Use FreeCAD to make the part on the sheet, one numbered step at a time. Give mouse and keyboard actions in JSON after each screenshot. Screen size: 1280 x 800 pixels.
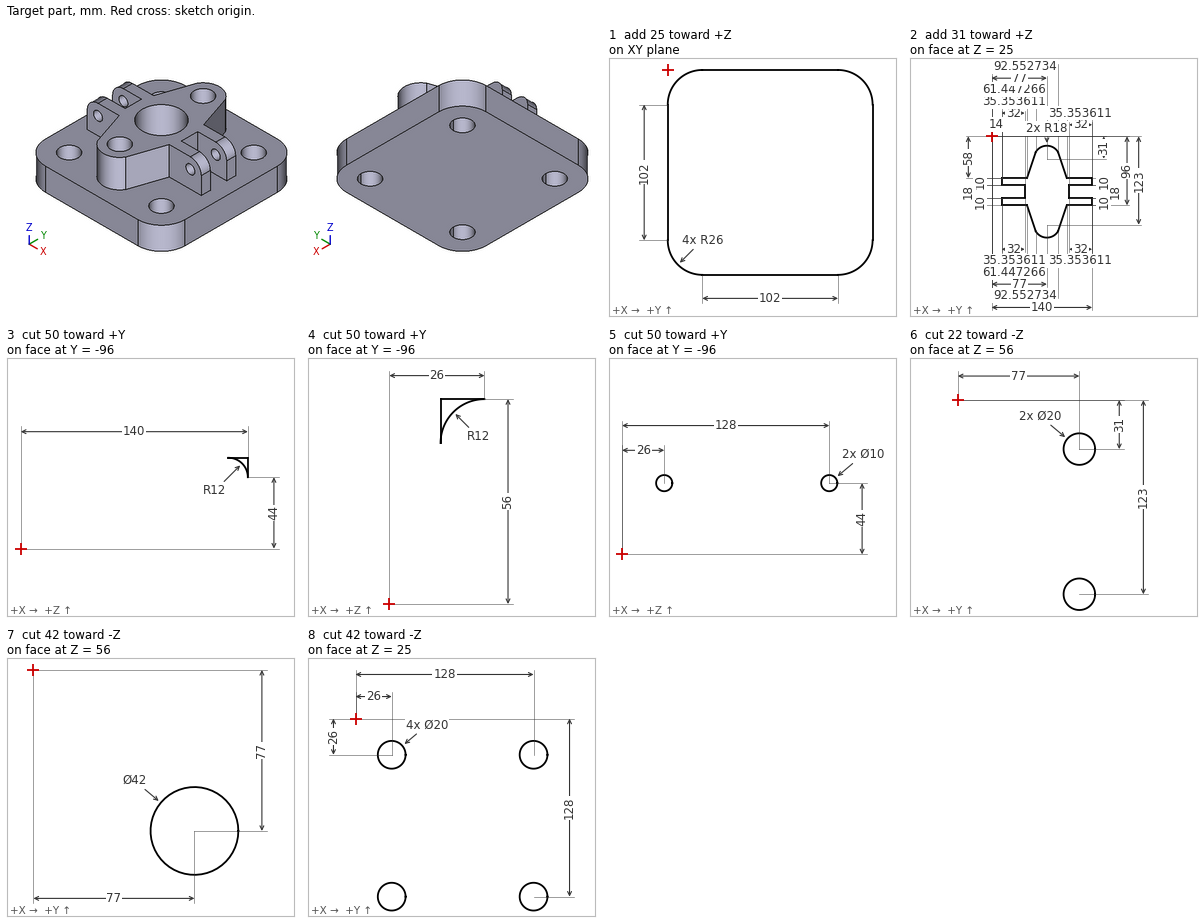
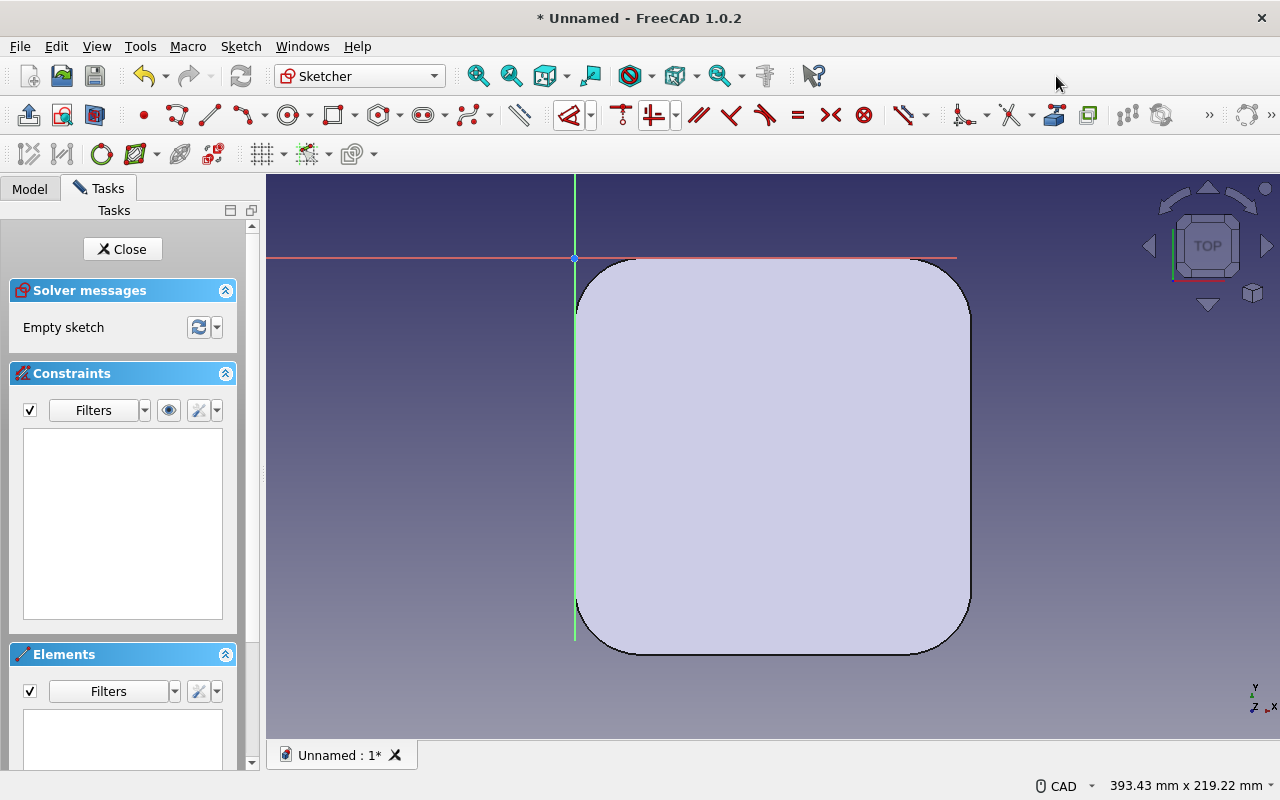
{"action": "left_click", "coordinate": [177, 116]}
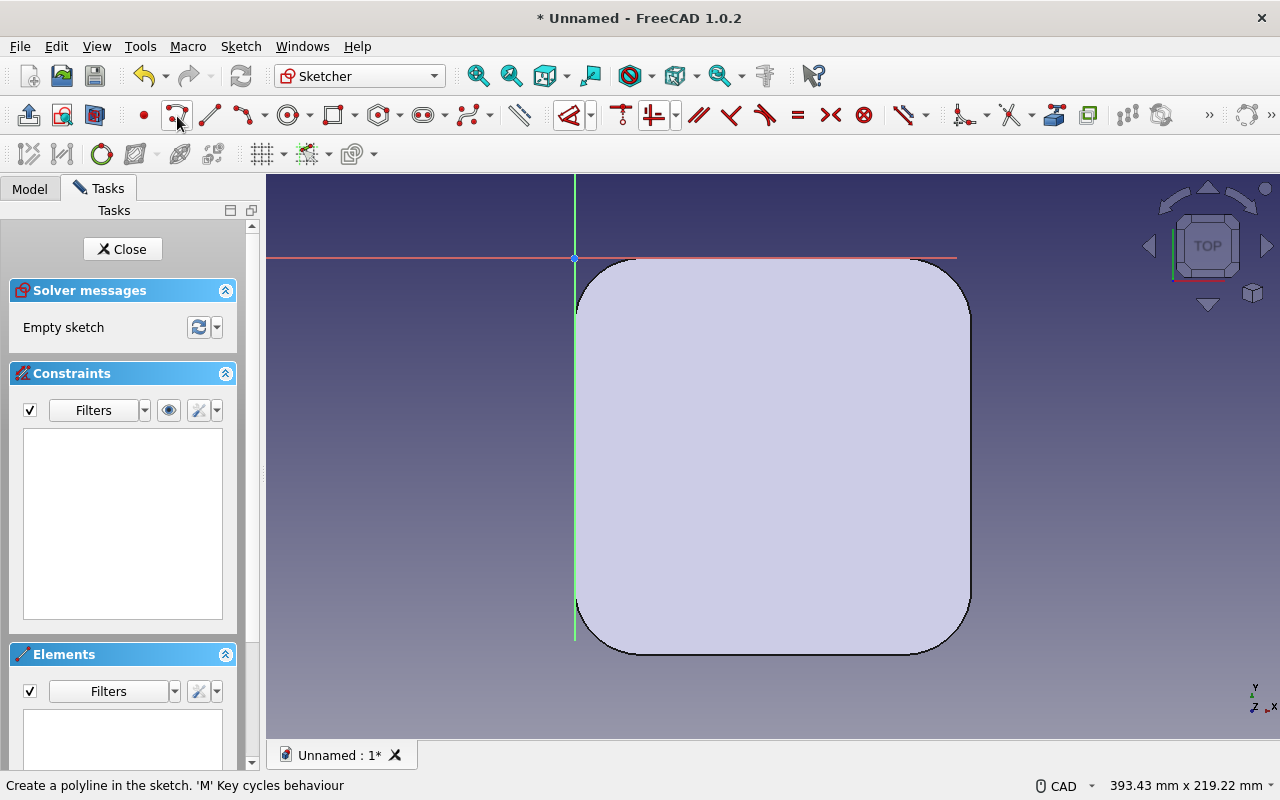
{"action": "left_click", "coordinate": [813, 598]}
{"action": "left_click", "coordinate": [844, 505]}
{"action": "left_click", "coordinate": [935, 505]}
{"action": "left_click", "coordinate": [935, 480]}
{"action": "left_click", "coordinate": [853, 480]}
{"action": "left_click", "coordinate": [853, 433]}
{"action": "left_click", "coordinate": [935, 433]}
{"action": "left_click", "coordinate": [935, 408]}
{"action": "left_click", "coordinate": [844, 408]}
{"action": "left_click", "coordinate": [813, 315]}
{"action": "right_click", "coordinate": [813, 315]}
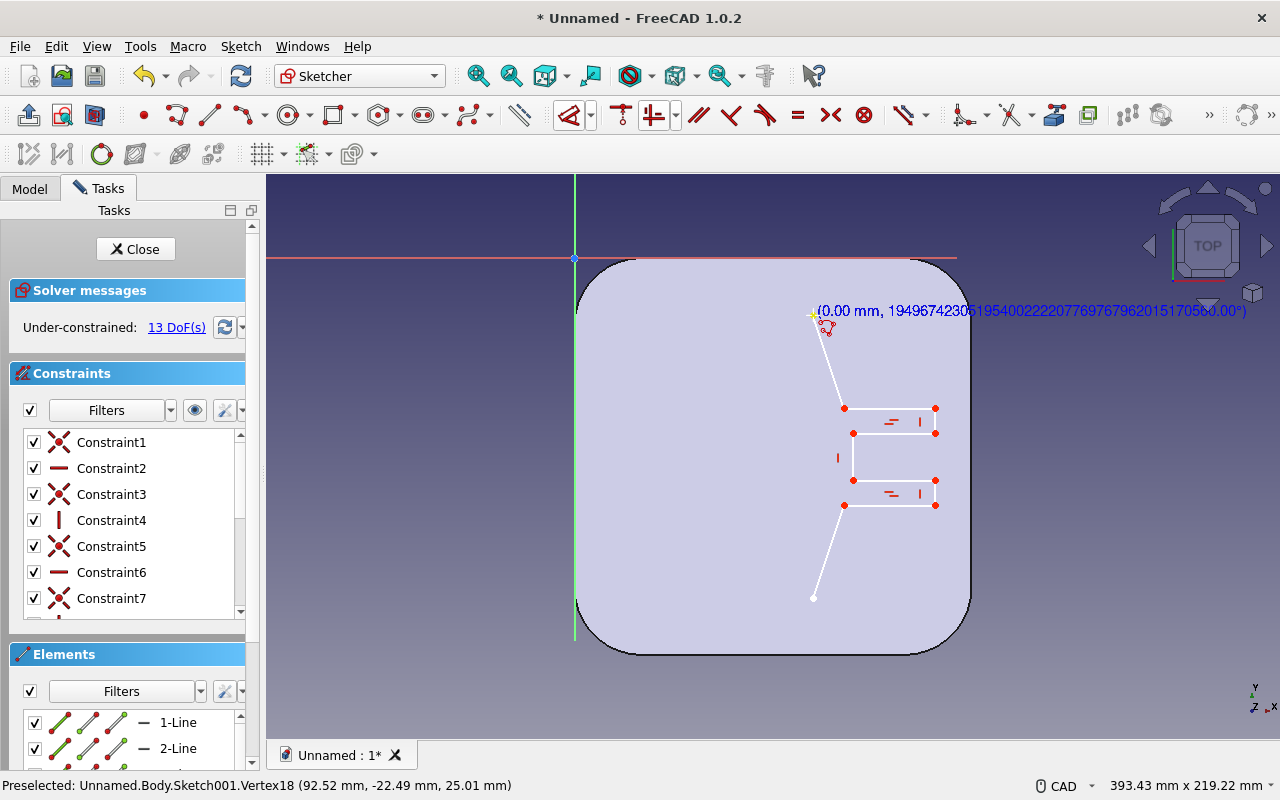
{"action": "left_click", "coordinate": [733, 315]}
{"action": "left_click", "coordinate": [702, 408]}
{"action": "left_click", "coordinate": [611, 408]}
{"action": "left_click", "coordinate": [611, 433]}
{"action": "left_click", "coordinate": [693, 433]}
{"action": "left_click", "coordinate": [693, 480]}
{"action": "left_click", "coordinate": [611, 480]}
{"action": "left_click", "coordinate": [611, 505]}
{"action": "left_click", "coordinate": [702, 505]}
{"action": "left_click", "coordinate": [733, 598]}
{"action": "right_click", "coordinate": [733, 598]}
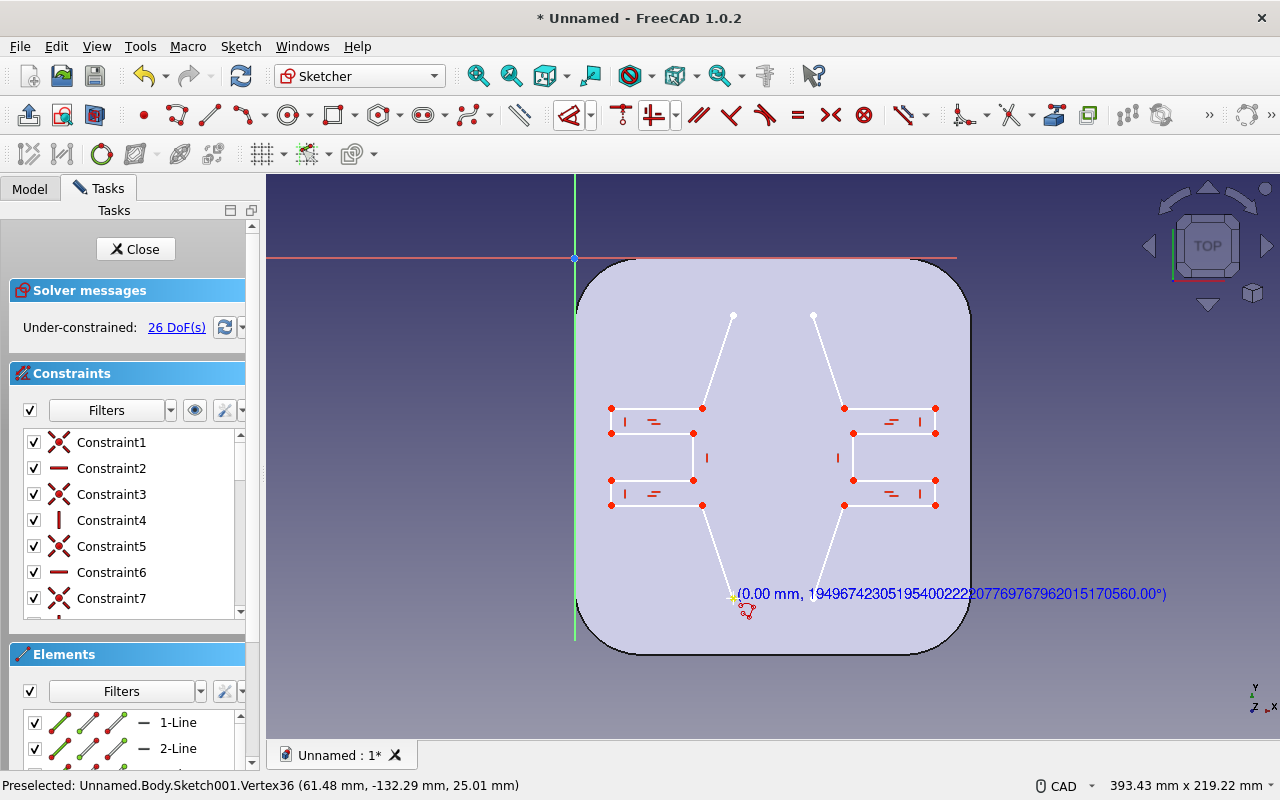
{"action": "left_click", "coordinate": [242, 116]}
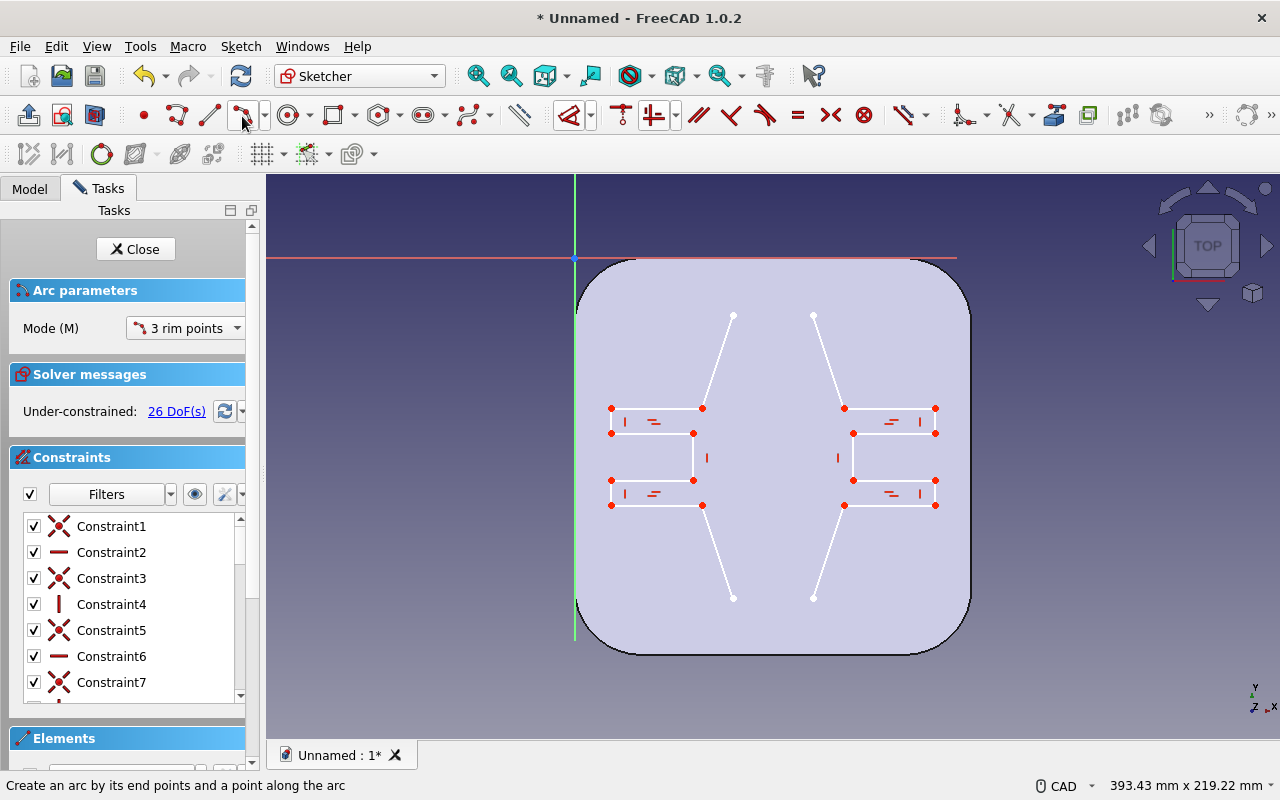
{"action": "left_click", "coordinate": [813, 316]}
{"action": "left_click", "coordinate": [733, 316]}
{"action": "left_click", "coordinate": [773, 292]}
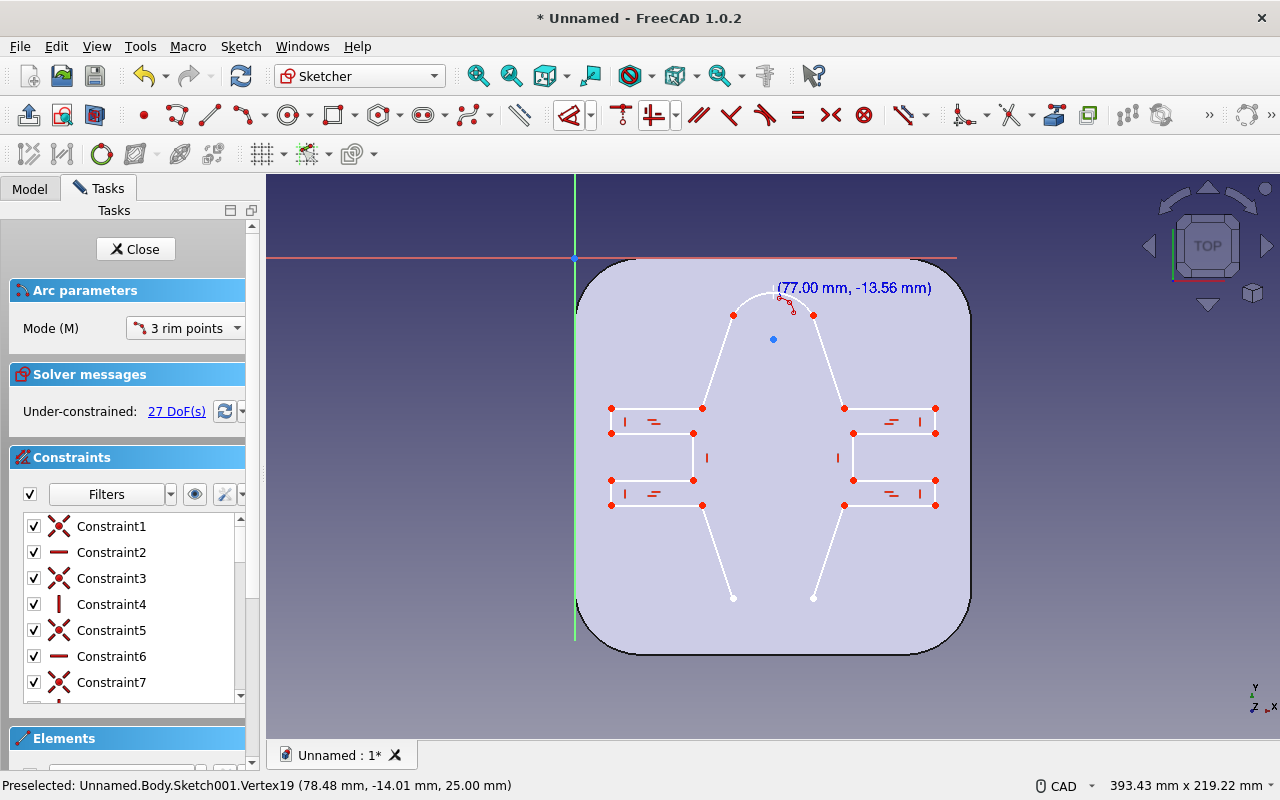
{"action": "left_click", "coordinate": [733, 599]}
{"action": "left_click", "coordinate": [813, 599]}
{"action": "left_click", "coordinate": [773, 621]}
{"action": "key", "text": "Escape"}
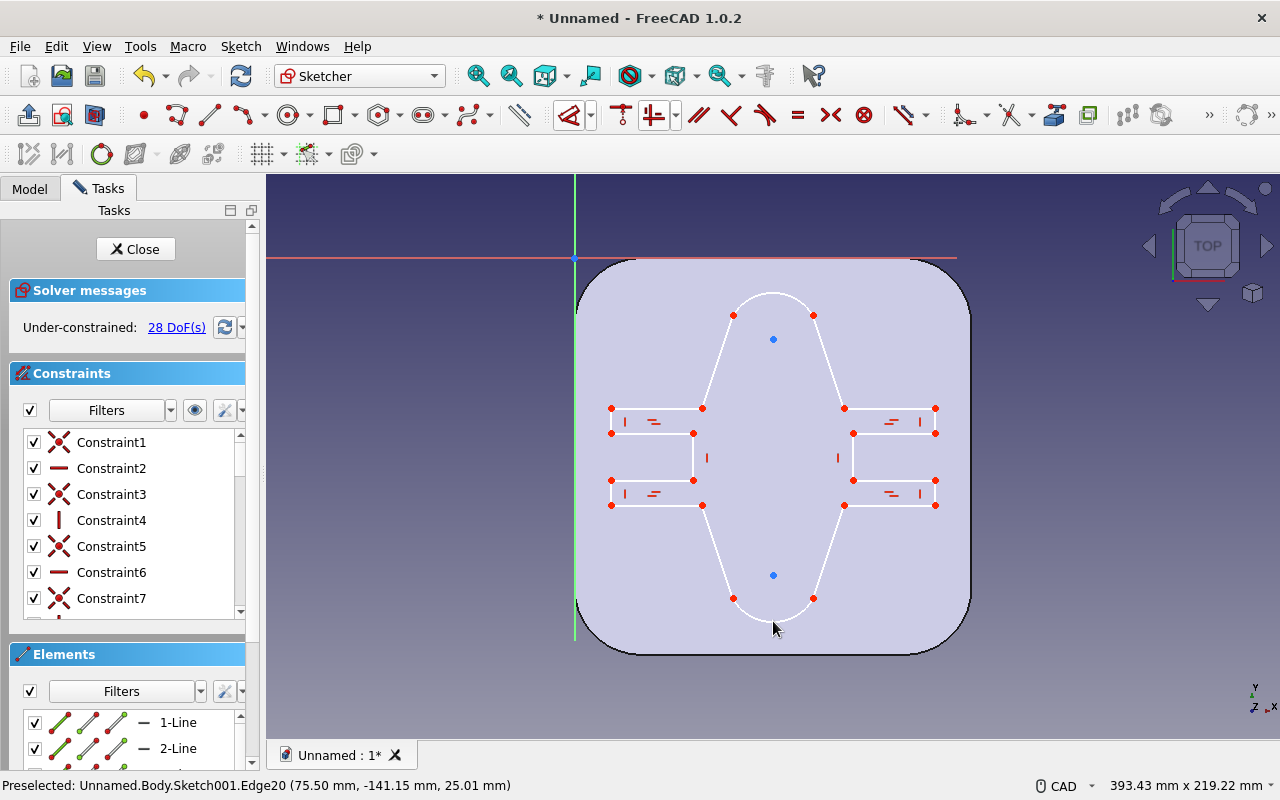
{"action": "left_click", "coordinate": [792, 297]}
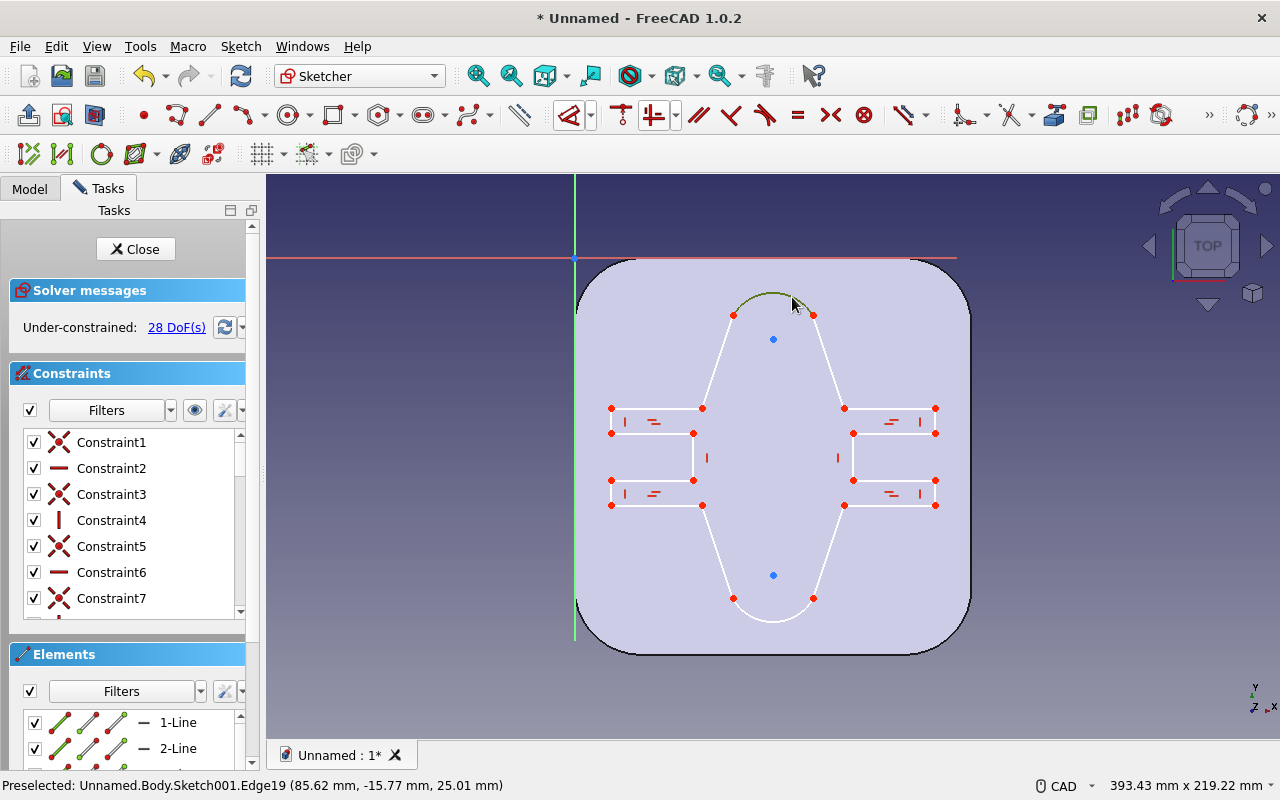
{"action": "left_click", "coordinate": [754, 618]}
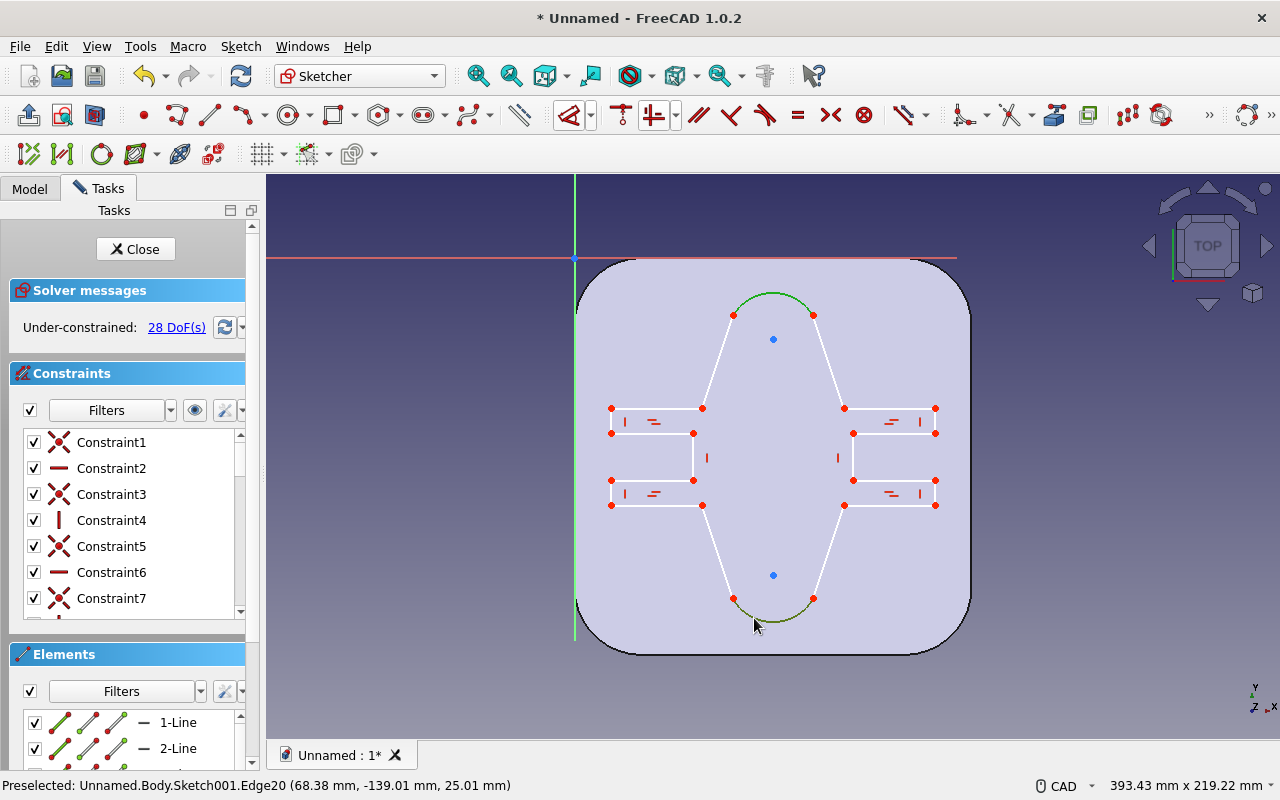
{"action": "left_click", "coordinate": [798, 116]}